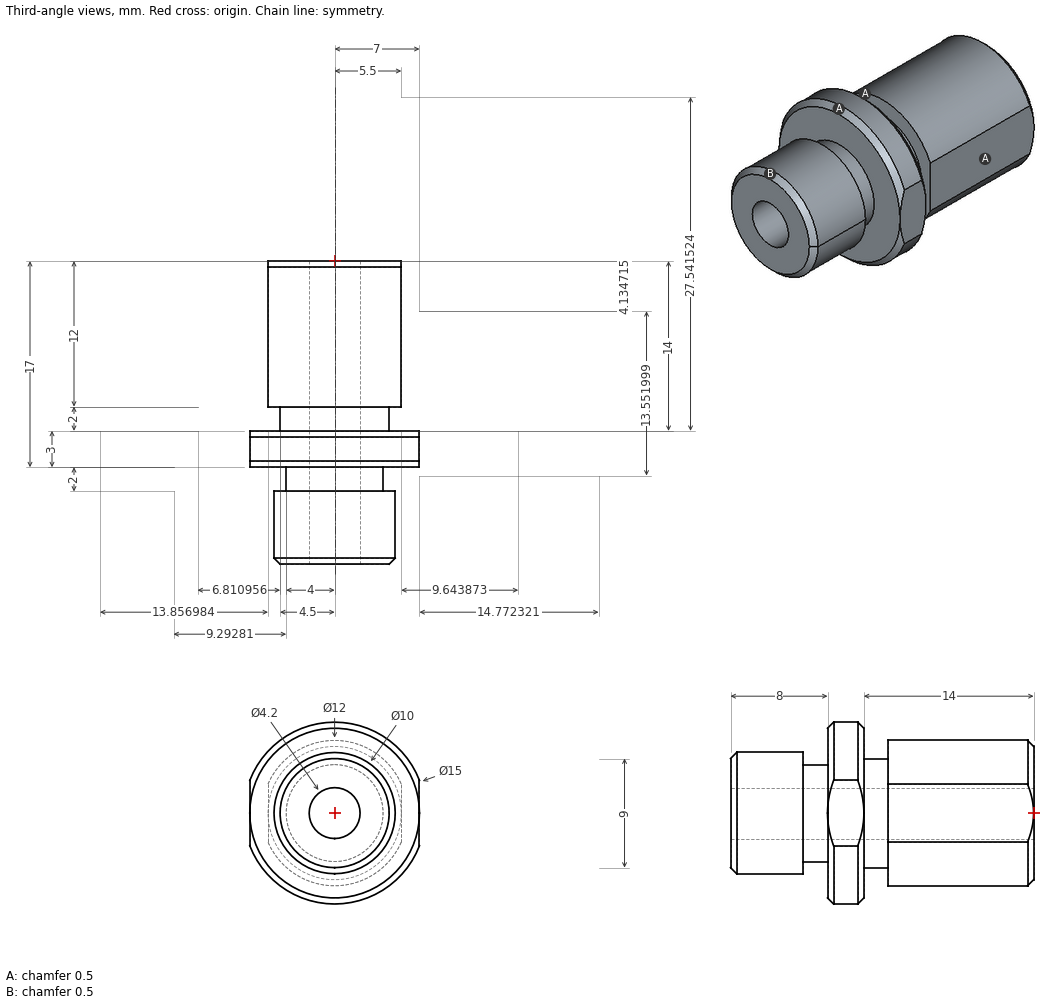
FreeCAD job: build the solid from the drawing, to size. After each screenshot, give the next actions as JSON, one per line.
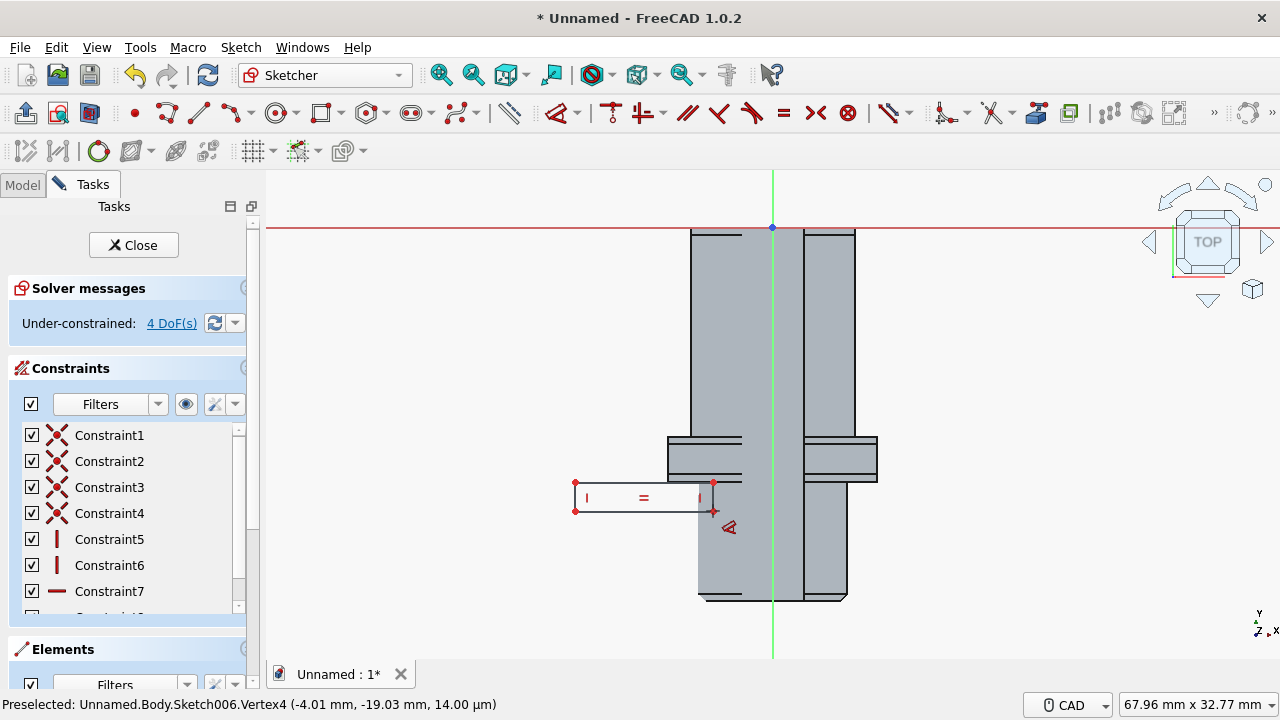
{"action": "scroll", "coordinate": [575, 495], "scroll_direction": "up", "scroll_amount": 2}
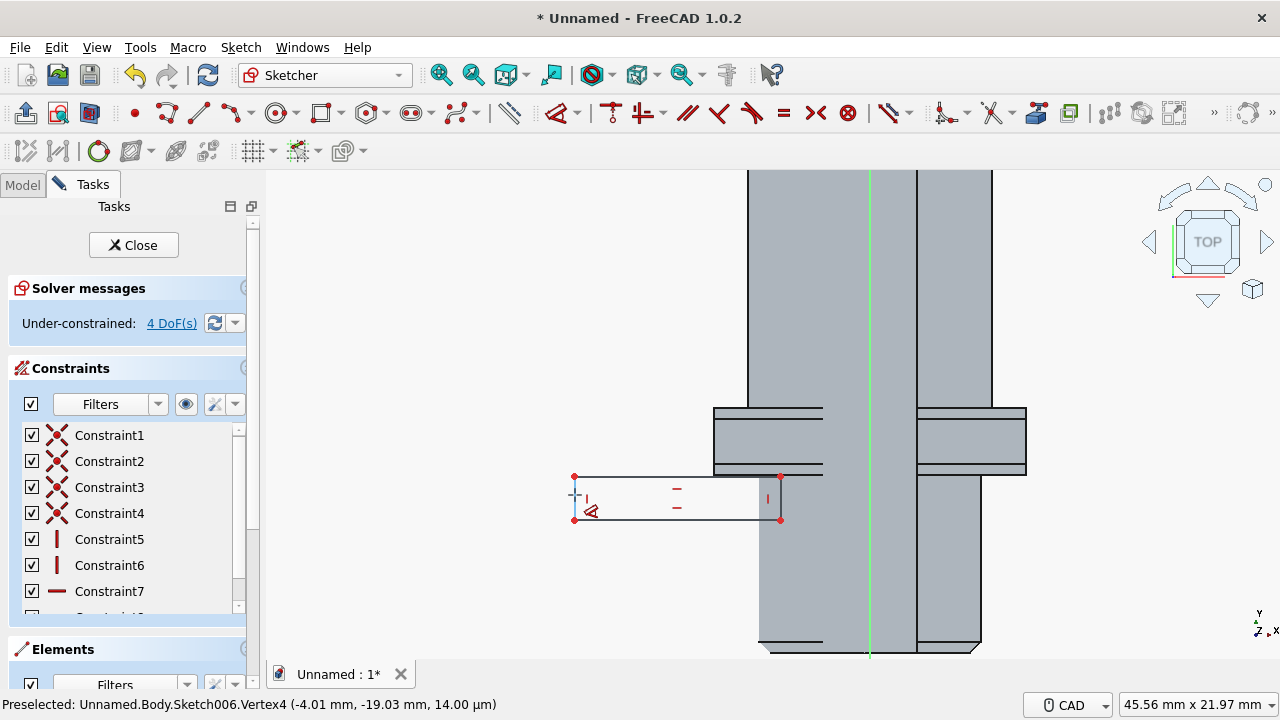
{"action": "left_click", "coordinate": [575, 494]}
{"action": "left_click", "coordinate": [541, 498]}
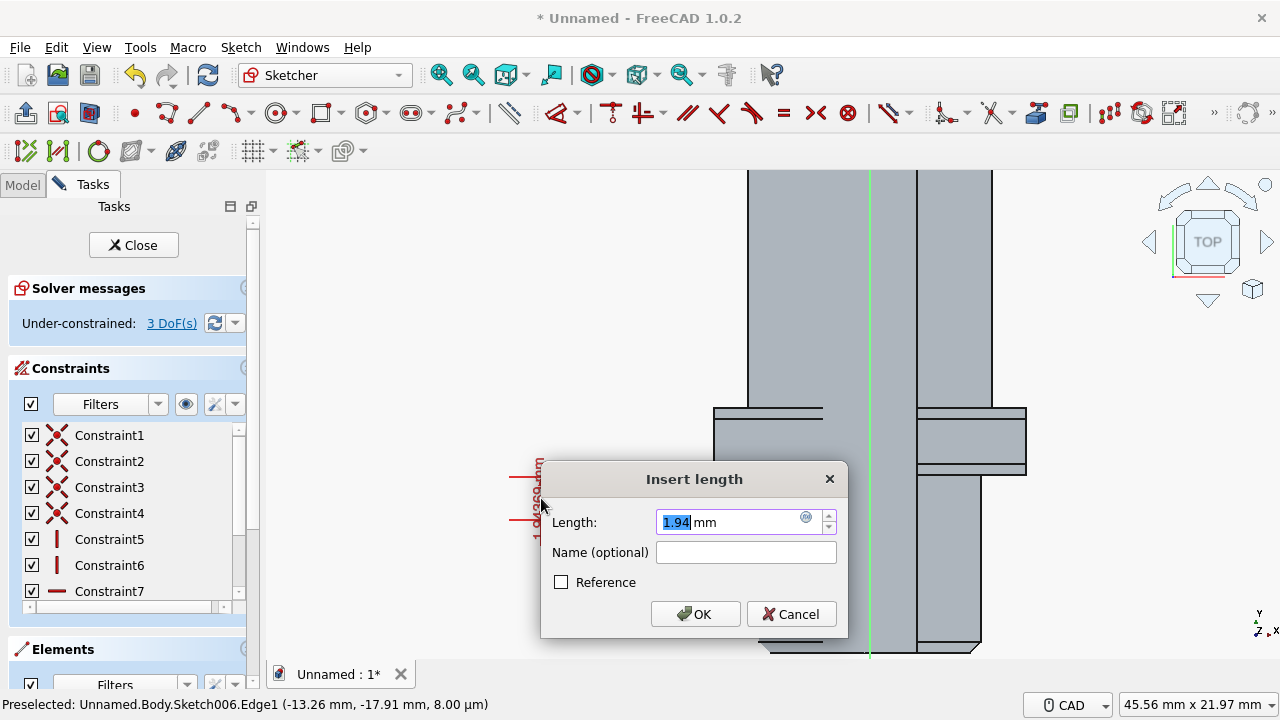
{"action": "type", "text": "2"}
{"action": "key", "text": "Return"}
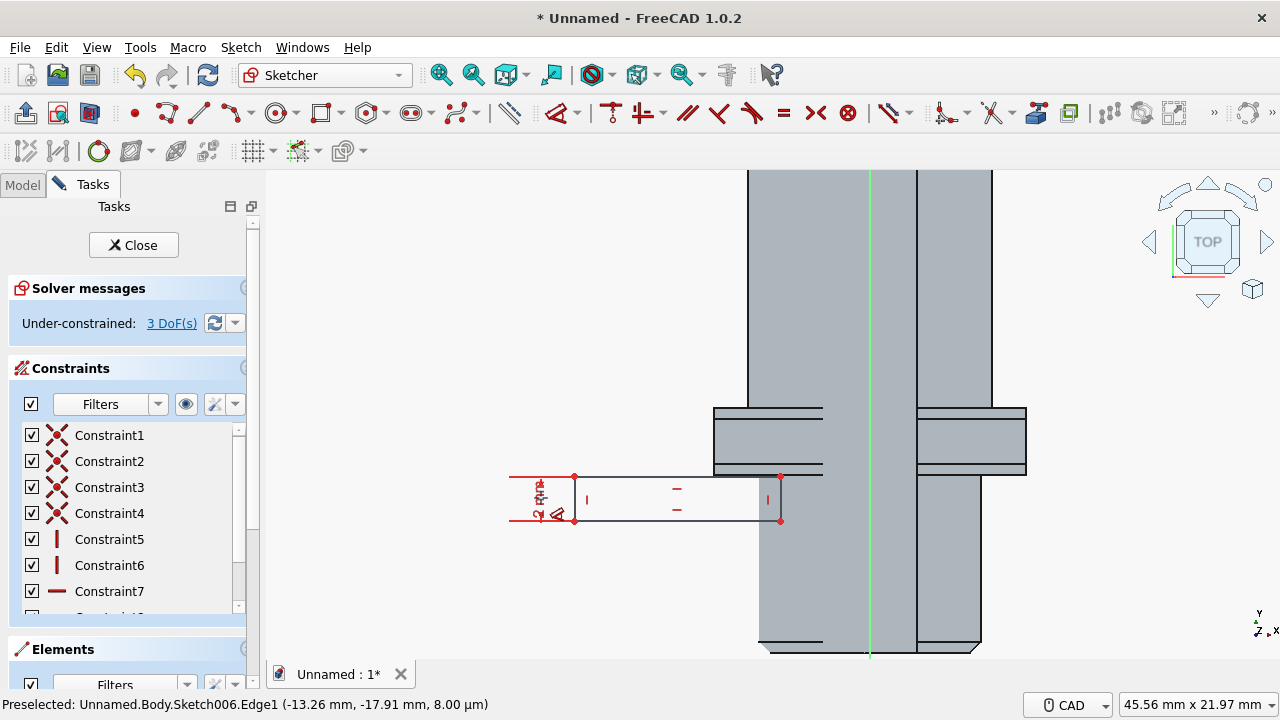
{"action": "left_click", "coordinate": [781, 521]}
{"action": "left_click", "coordinate": [825, 555]}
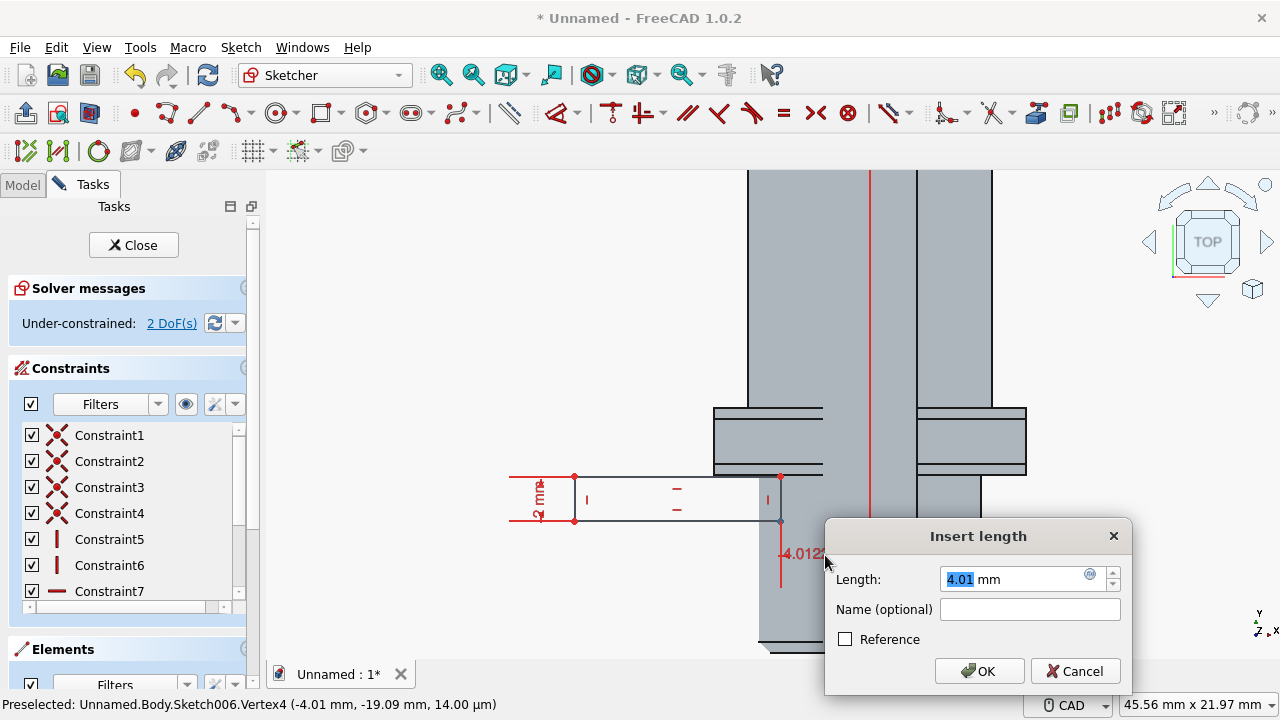
{"action": "type", "text": "4"}
{"action": "key", "text": "Return"}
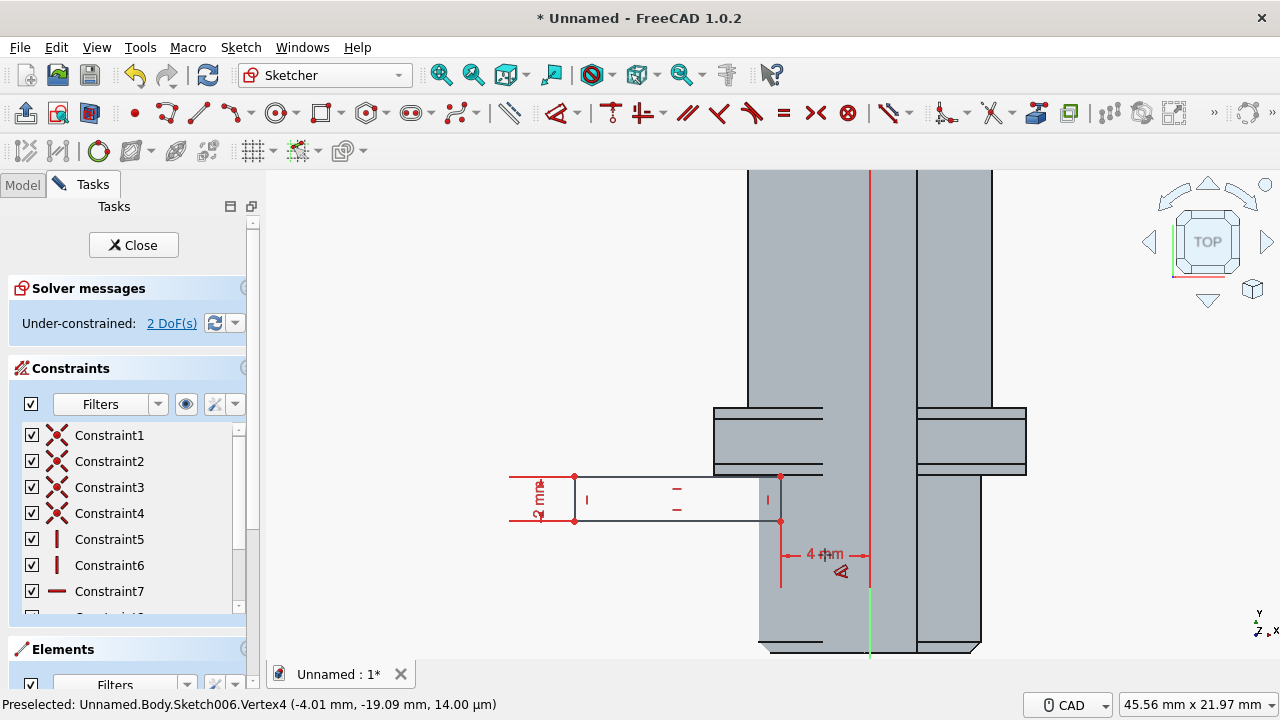
{"action": "left_click", "coordinate": [575, 477]}
{"action": "left_click", "coordinate": [904, 337]}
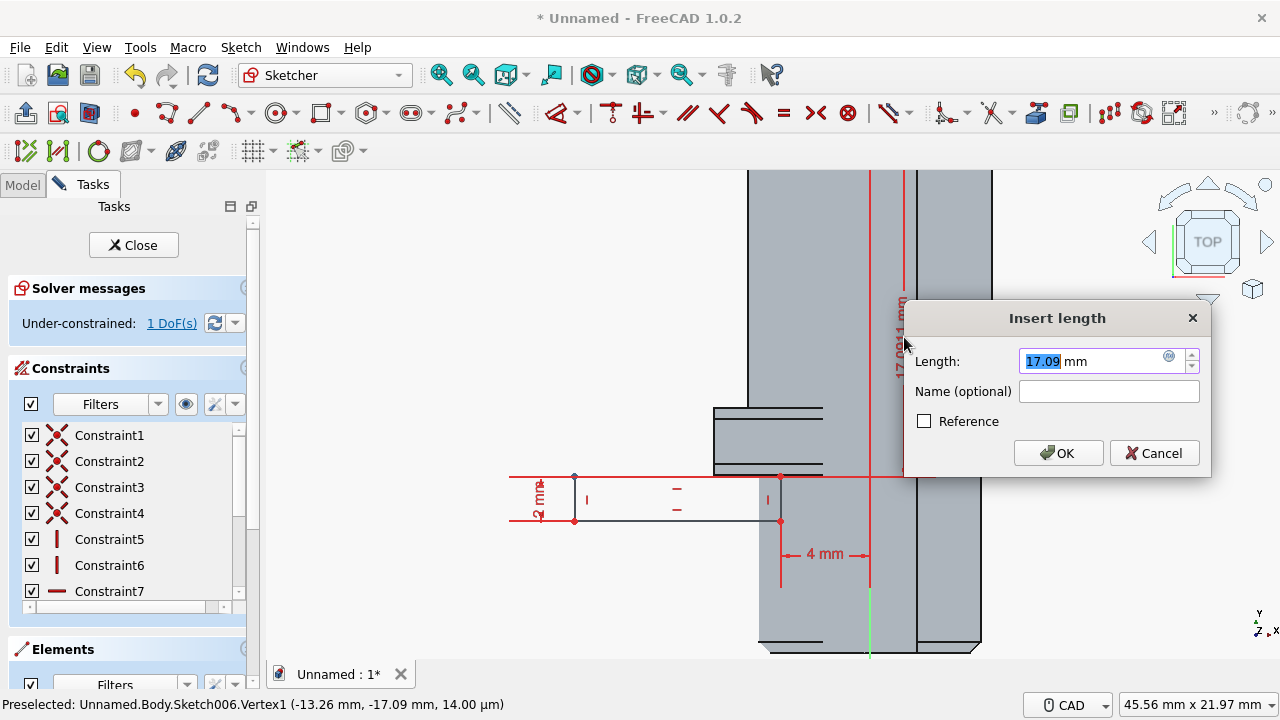
{"action": "type", "text": "17"}
{"action": "key", "text": "Return"}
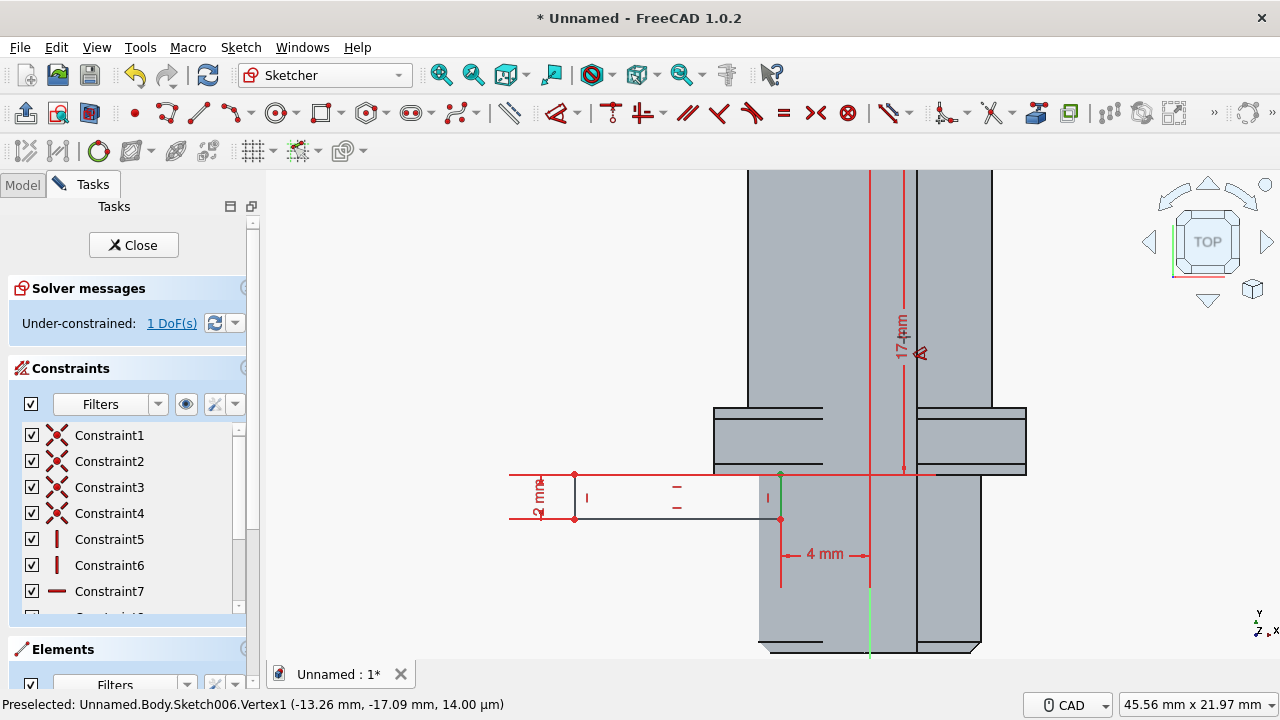
{"action": "left_click", "coordinate": [637, 519]}
{"action": "left_click", "coordinate": [678, 553]}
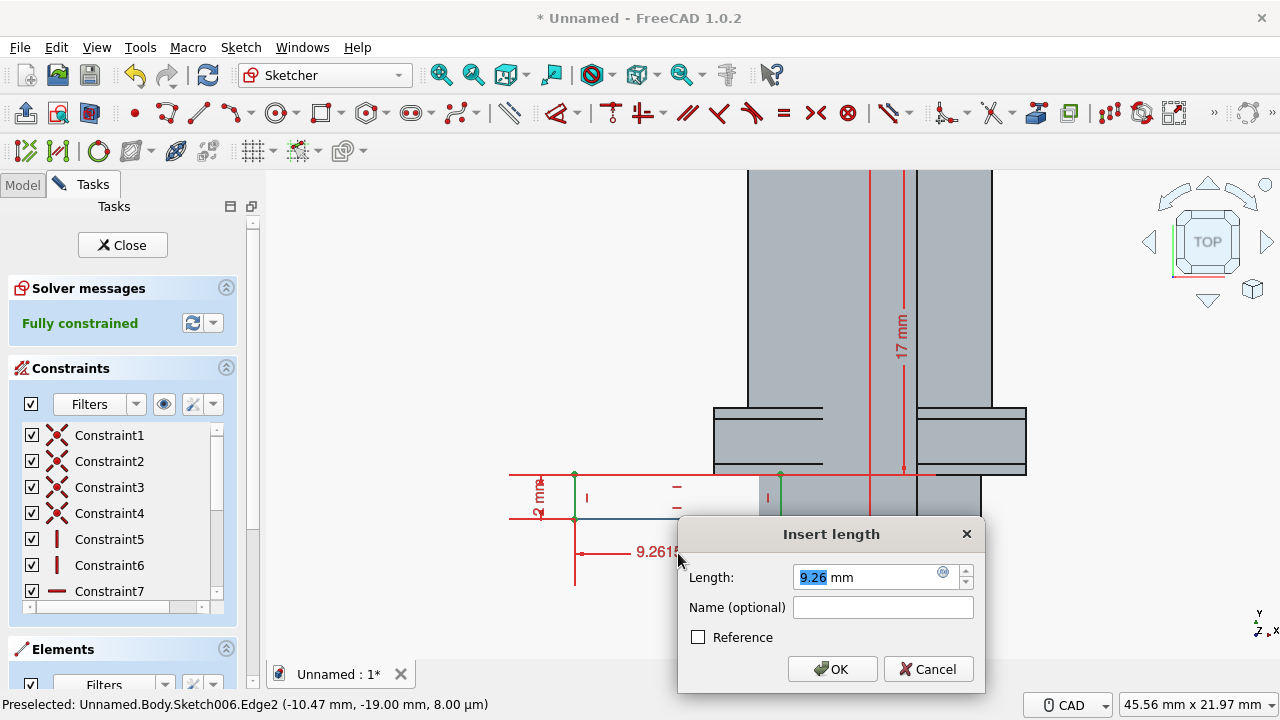
{"action": "type", "text": "9.29281"}
{"action": "key", "text": "Return"}
{"action": "key", "text": "Escape"}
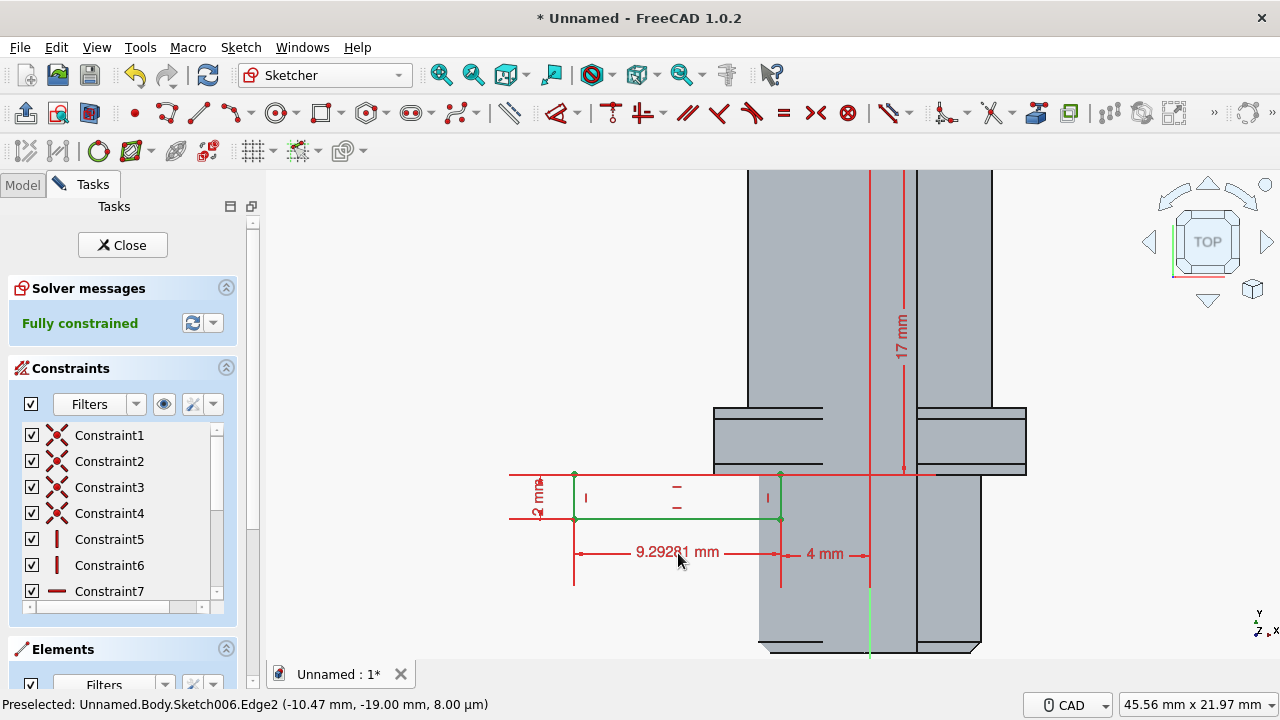
{"action": "left_click", "coordinate": [123, 245]}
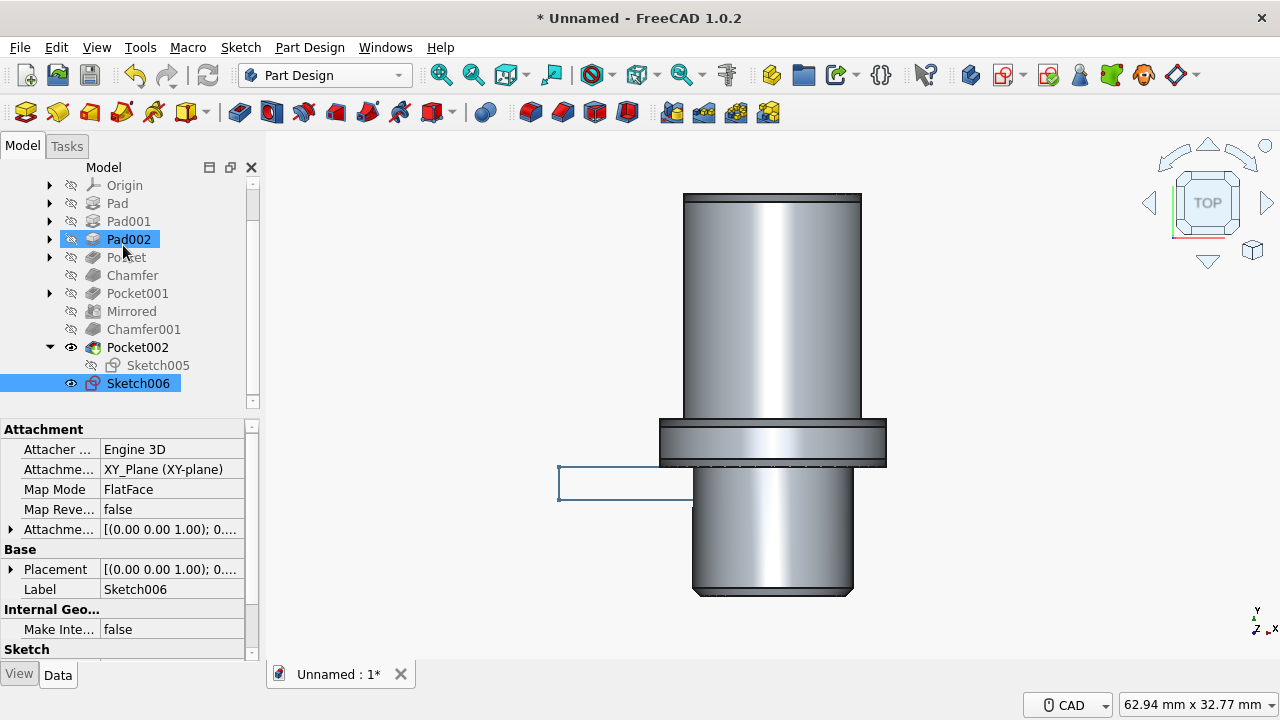
{"action": "left_click", "coordinate": [304, 112]}